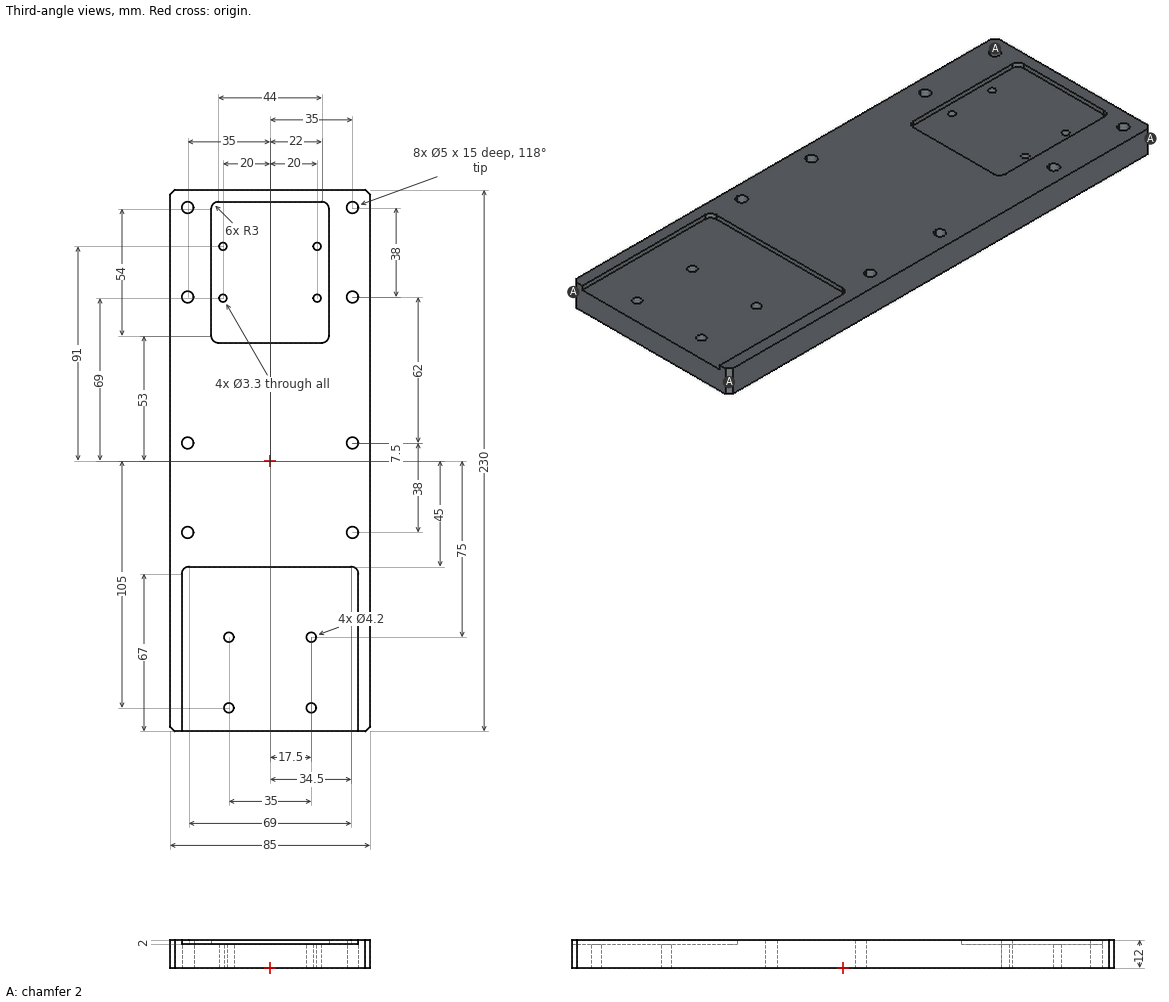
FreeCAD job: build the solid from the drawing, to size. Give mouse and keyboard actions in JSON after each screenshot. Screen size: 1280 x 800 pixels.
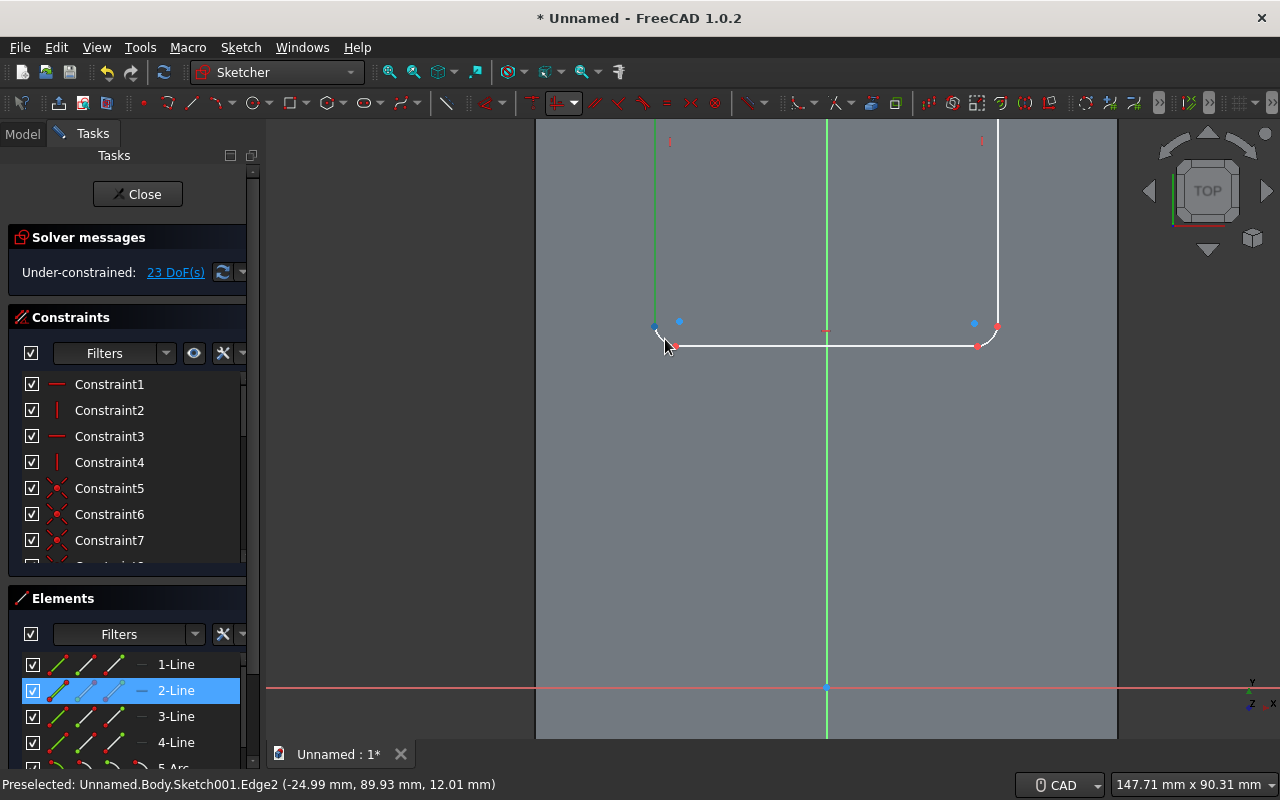
{"action": "left_click", "coordinate": [662, 340]}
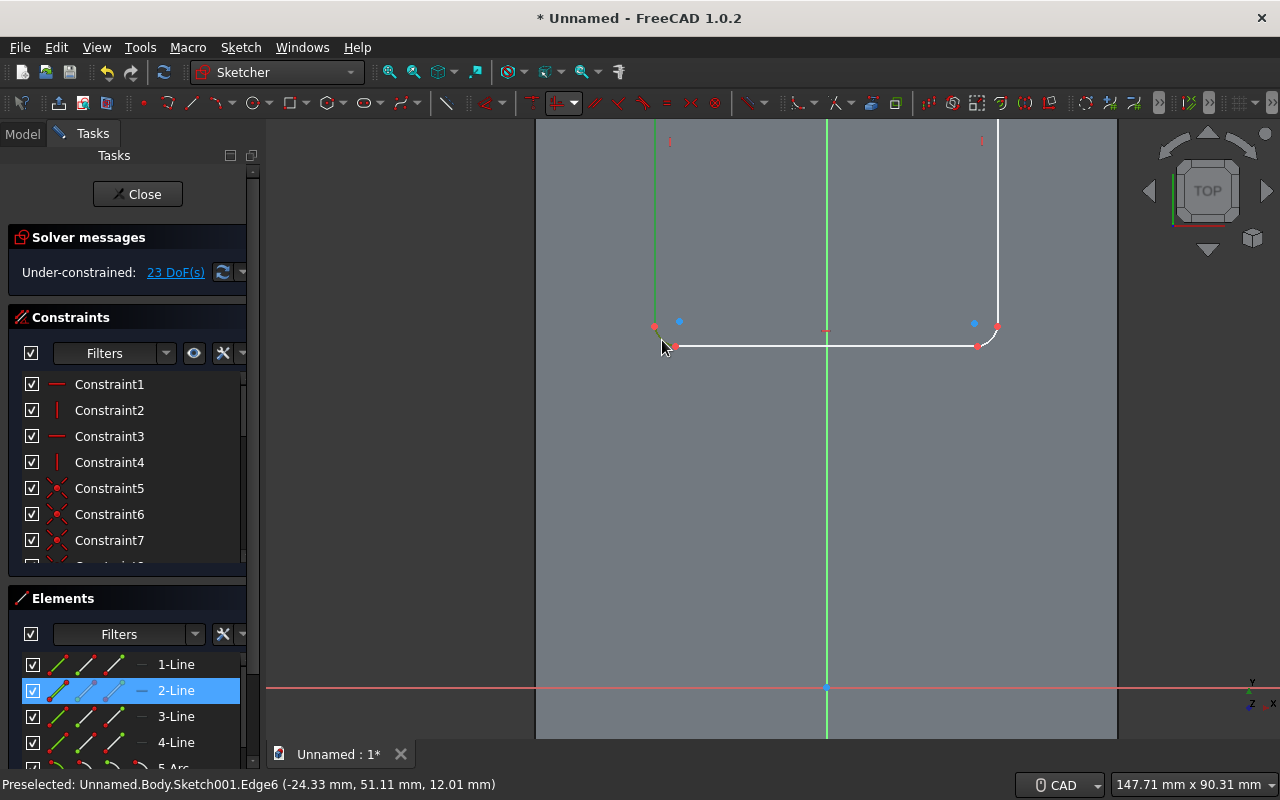
{"action": "key", "text": "t"}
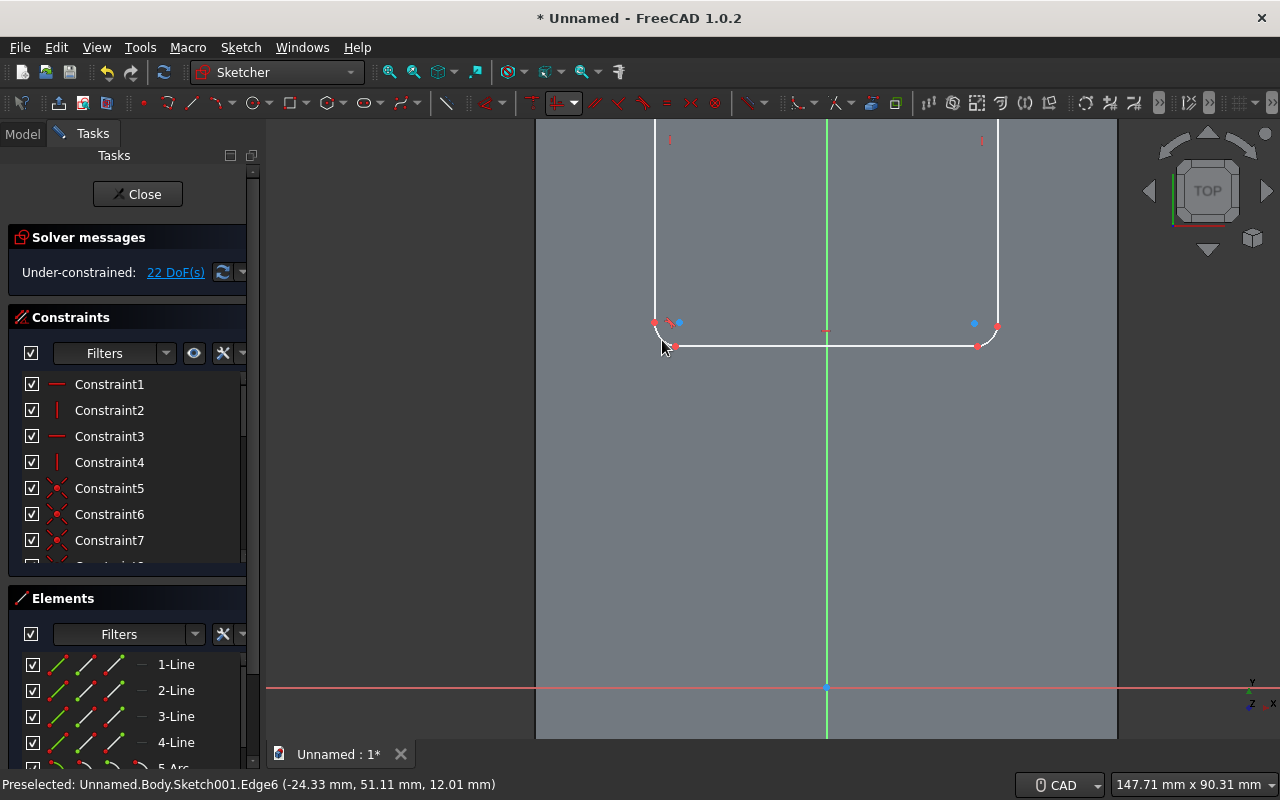
{"action": "scroll", "coordinate": [665, 339], "scroll_direction": "down", "scroll_amount": 7}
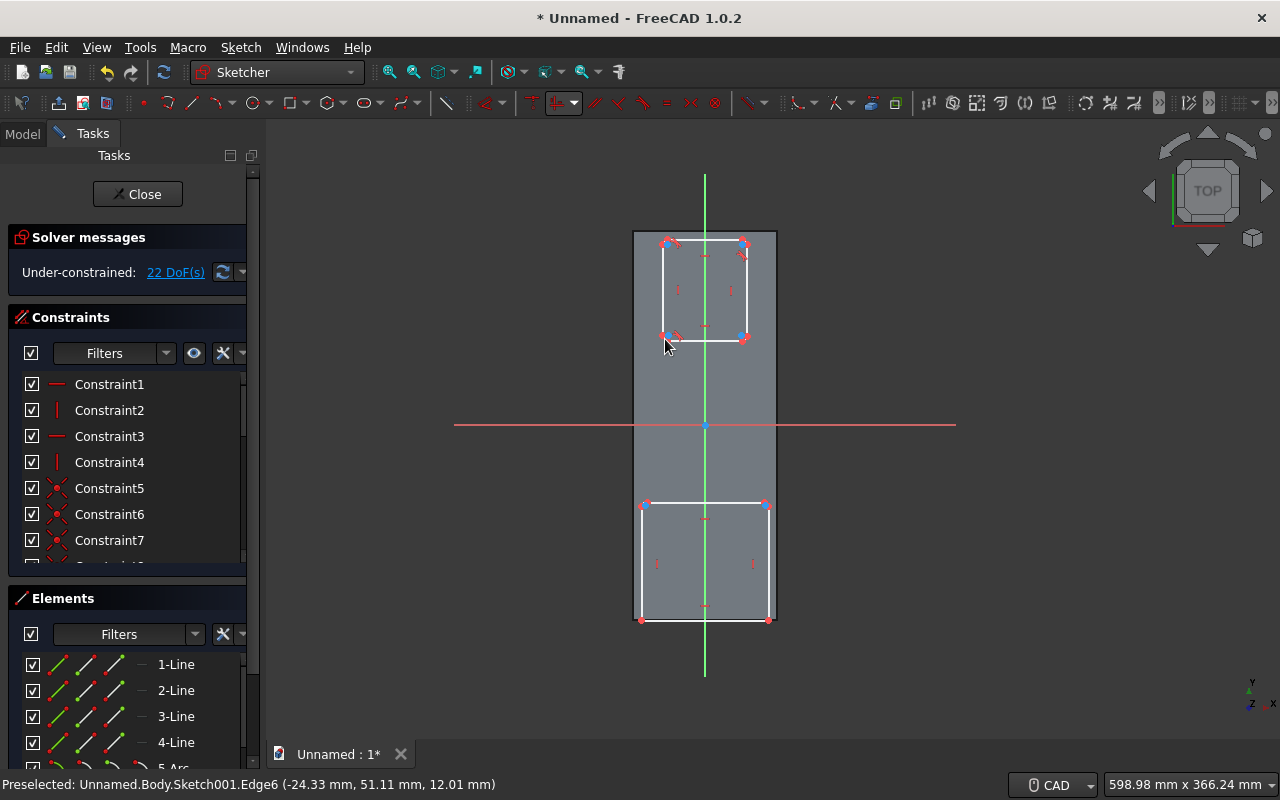
{"action": "left_click", "coordinate": [690, 341]}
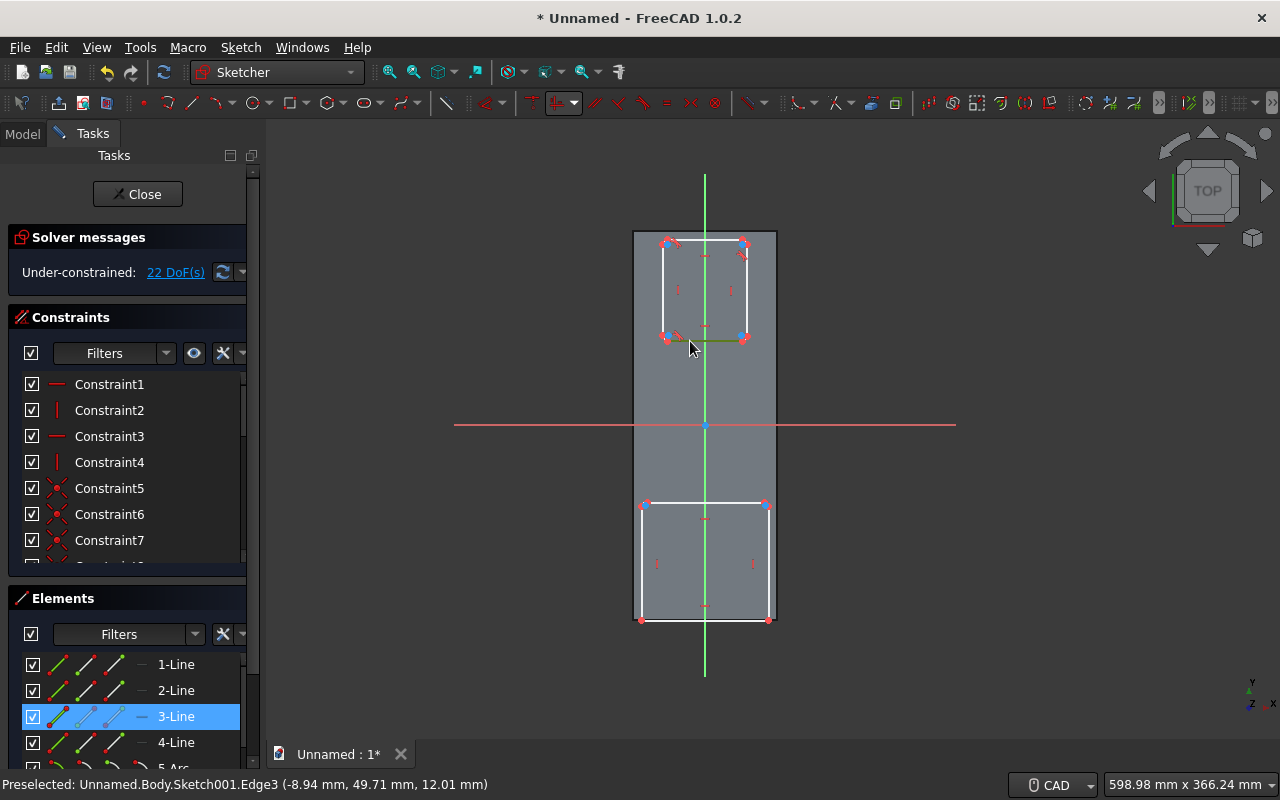
{"action": "scroll", "coordinate": [664, 339], "scroll_direction": "up", "scroll_amount": 7}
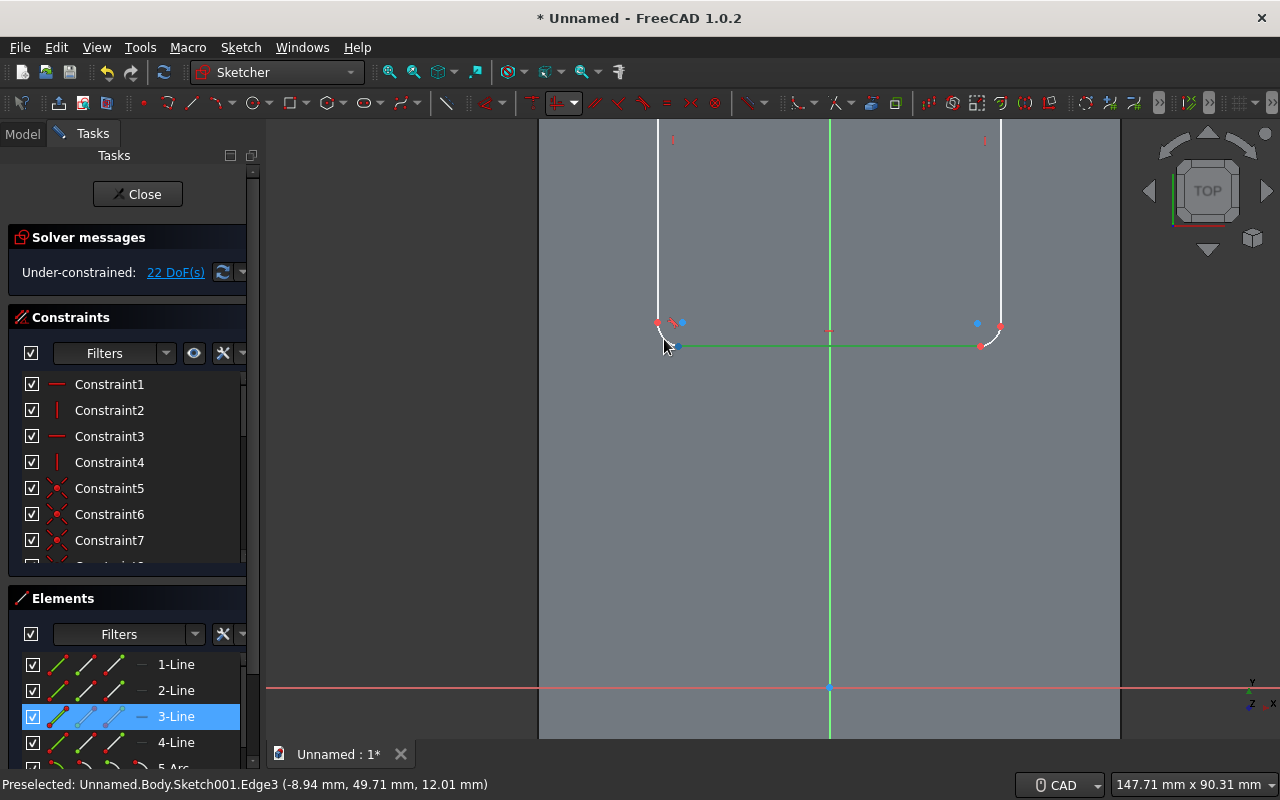
{"action": "left_click", "coordinate": [663, 338]}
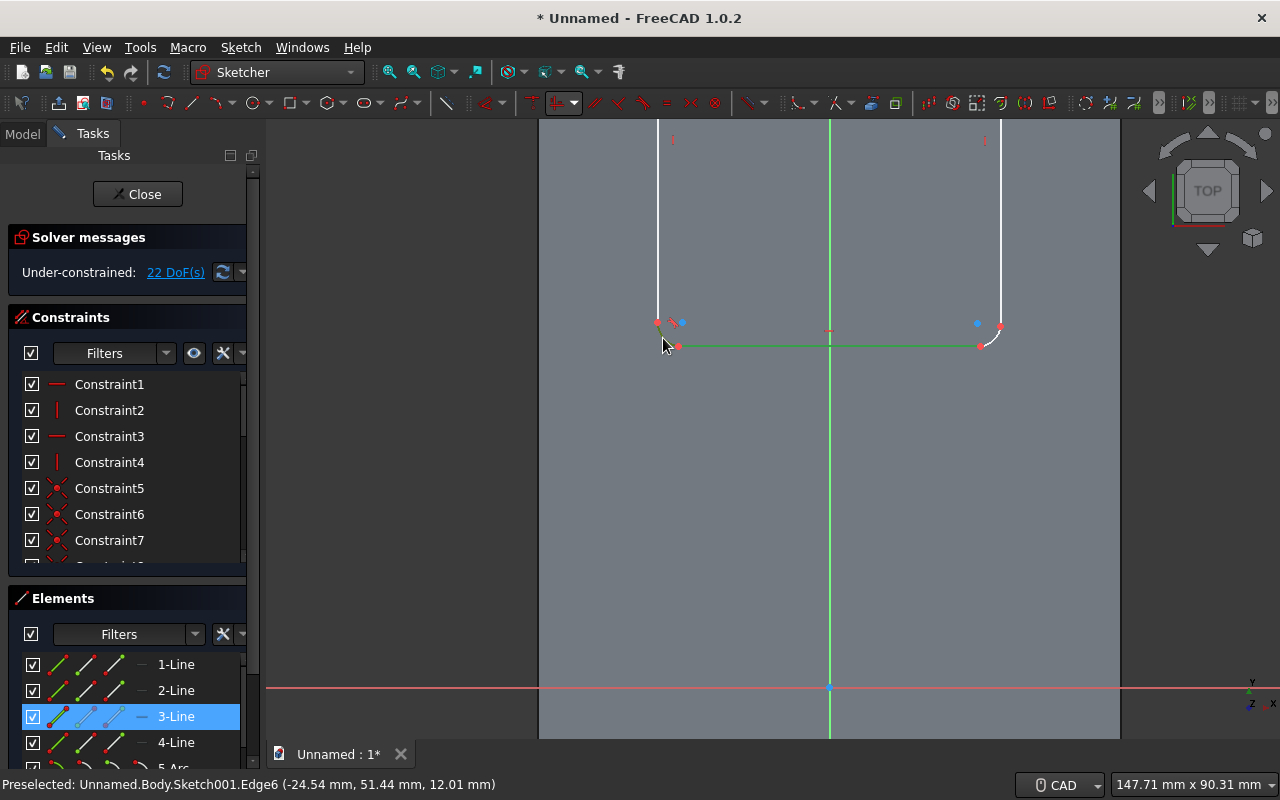
{"action": "left_click", "coordinate": [644, 104]}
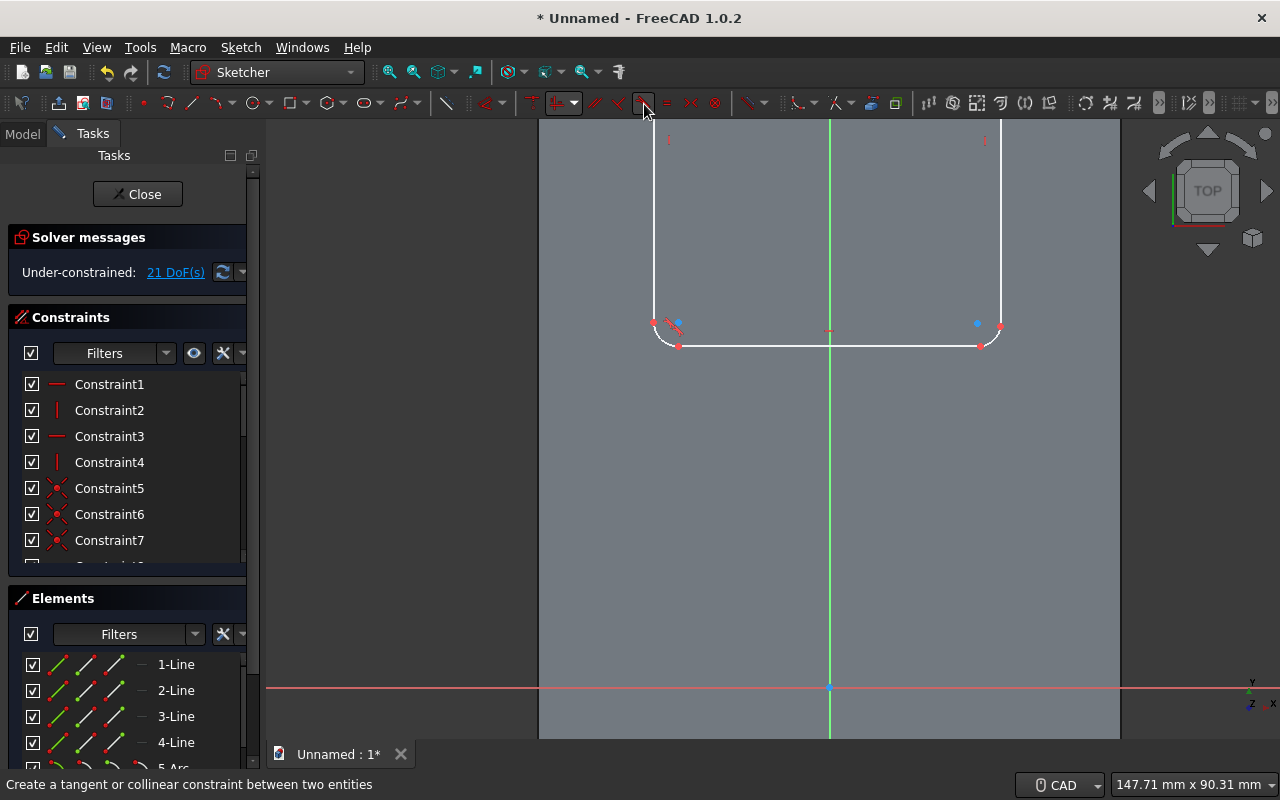
{"action": "scroll", "coordinate": [664, 339], "scroll_direction": "down", "scroll_amount": 7}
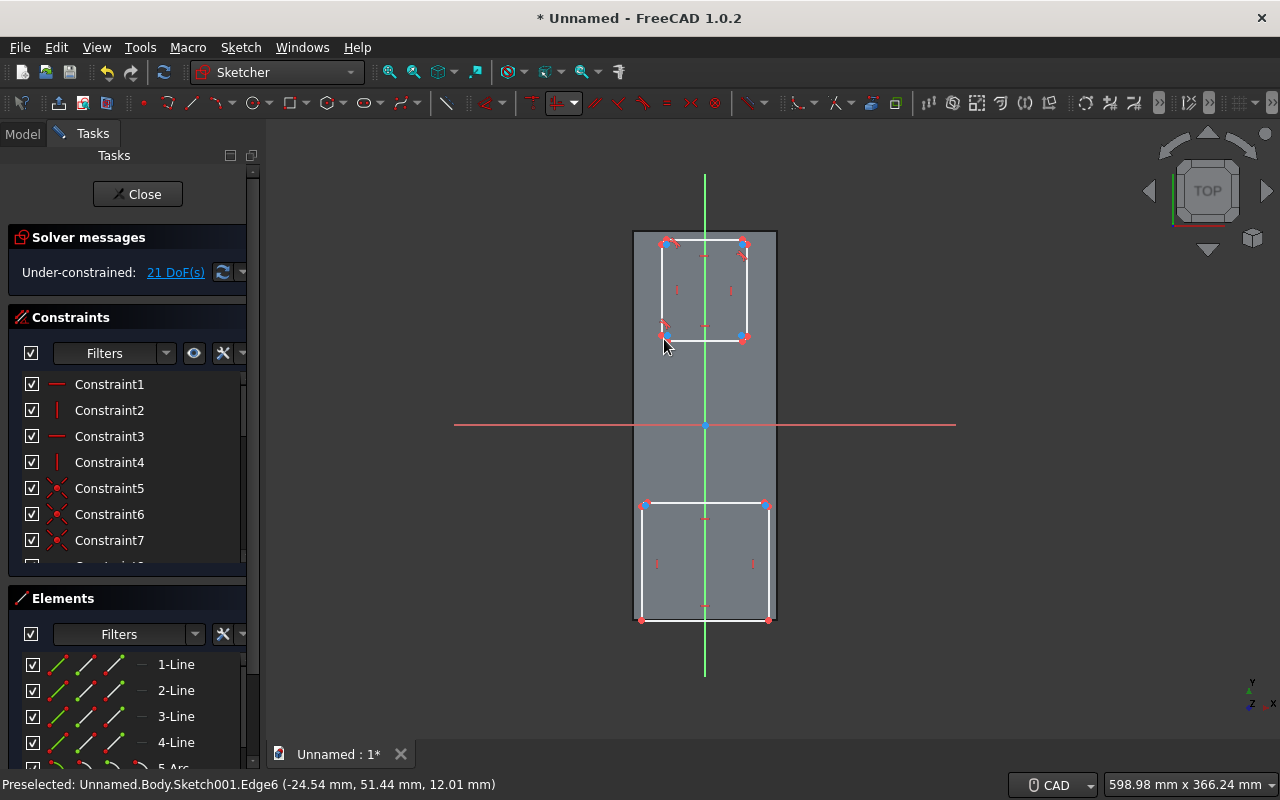
{"action": "left_click", "coordinate": [690, 341]}